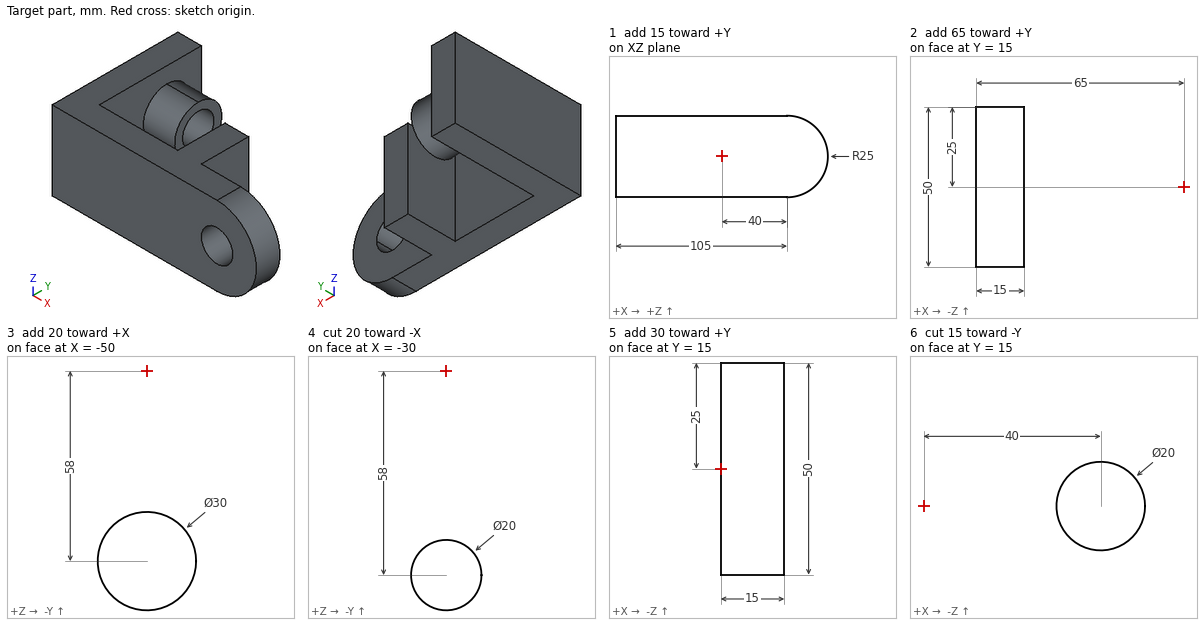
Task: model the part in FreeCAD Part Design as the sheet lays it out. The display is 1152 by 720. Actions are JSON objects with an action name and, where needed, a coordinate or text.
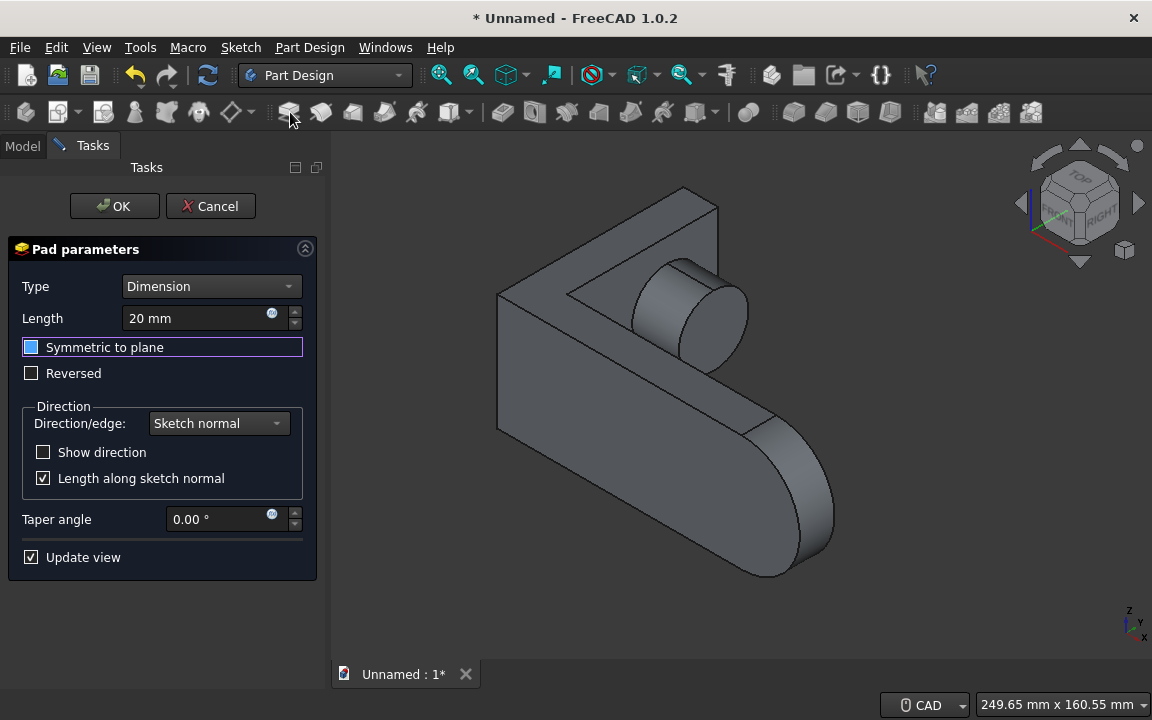
{"action": "left_click", "coordinate": [115, 206]}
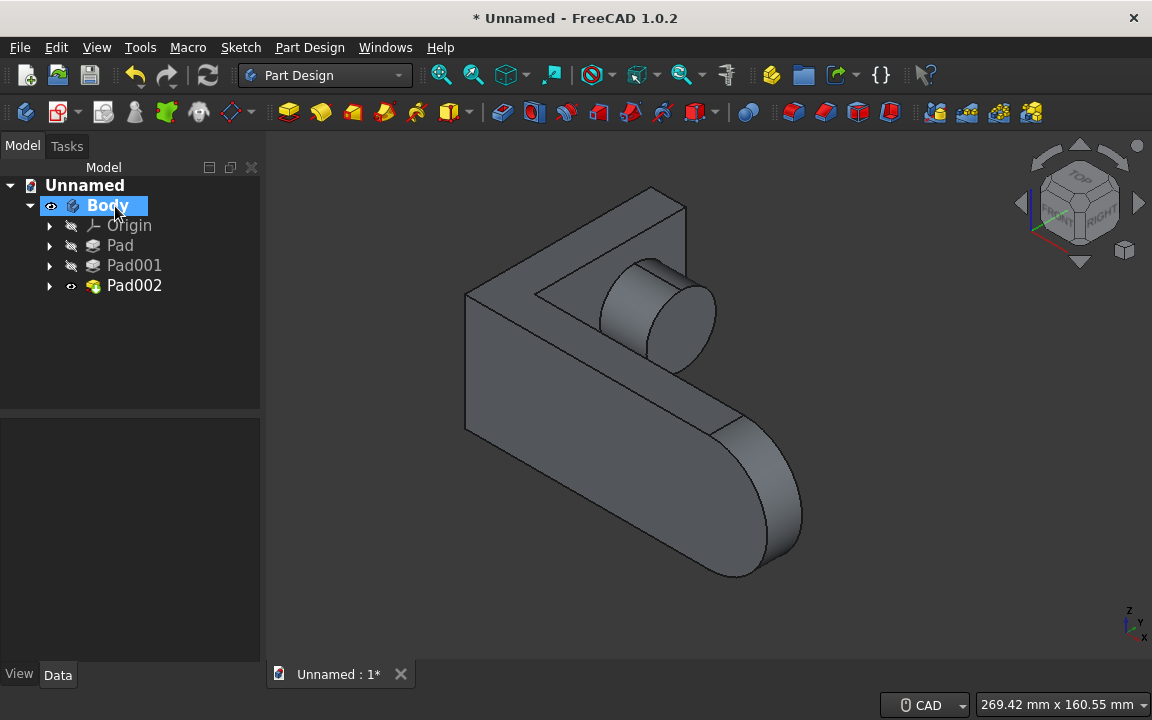
{"action": "left_click", "coordinate": [681, 330]}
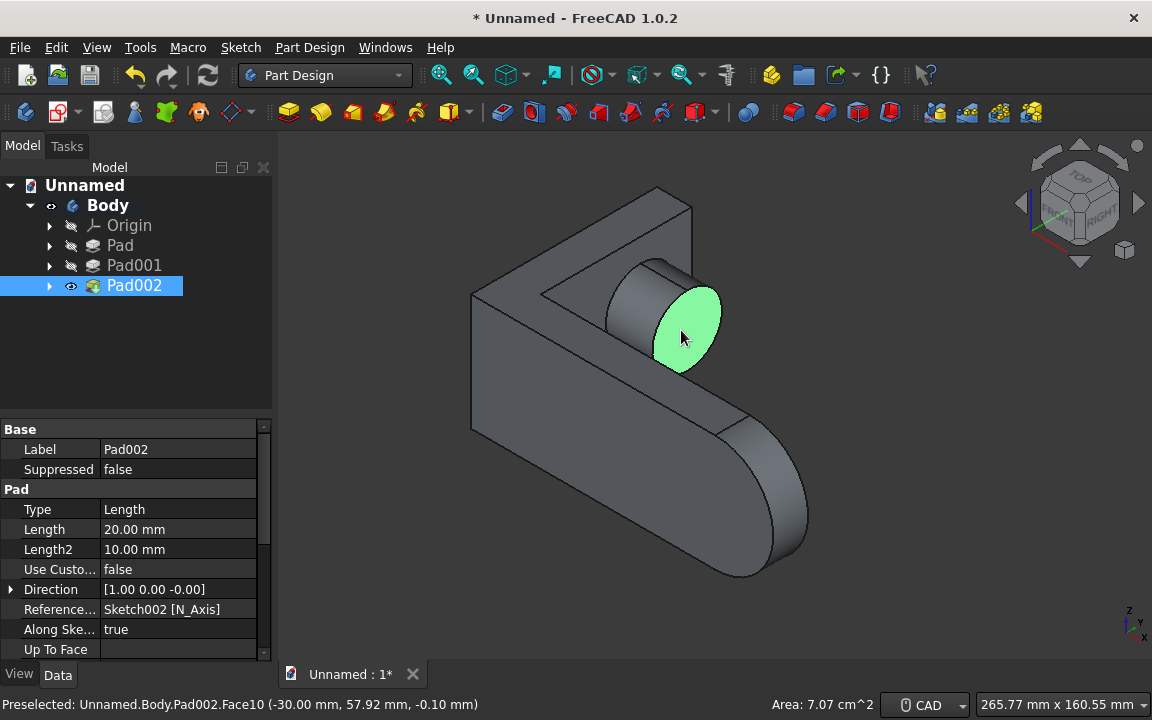
{"action": "left_click", "coordinate": [58, 112]}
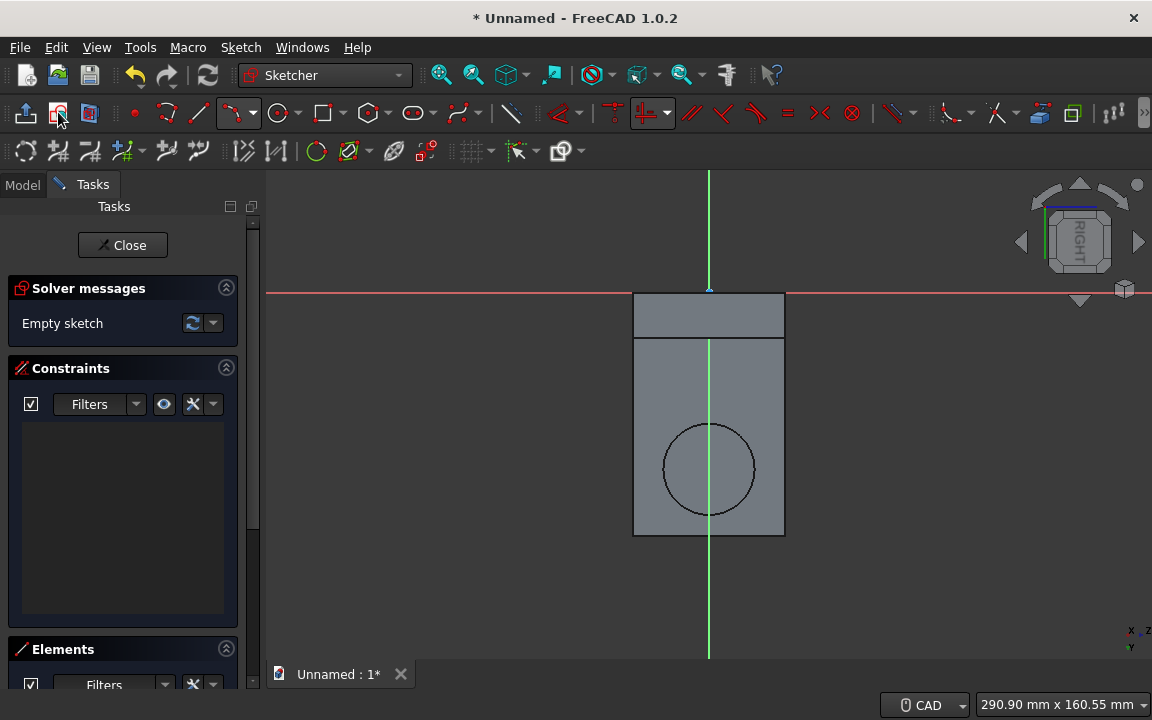
{"action": "left_click", "coordinate": [90, 114]}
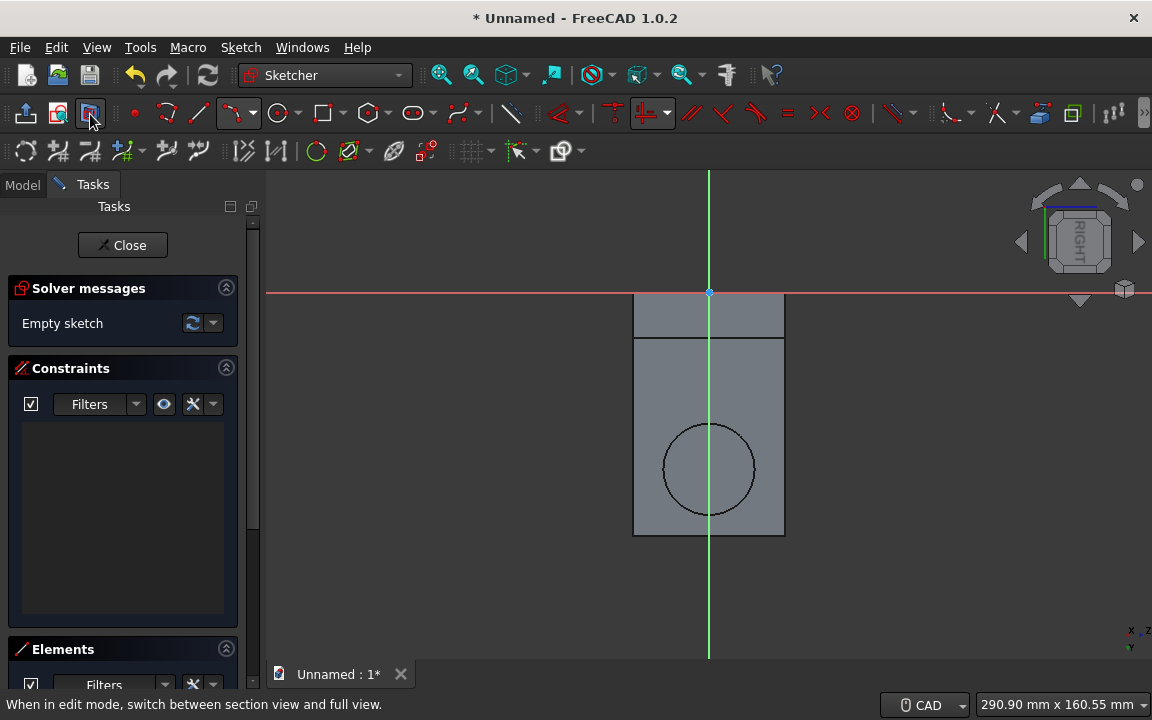
{"action": "scroll", "coordinate": [726, 483], "scroll_direction": "up", "scroll_amount": 8}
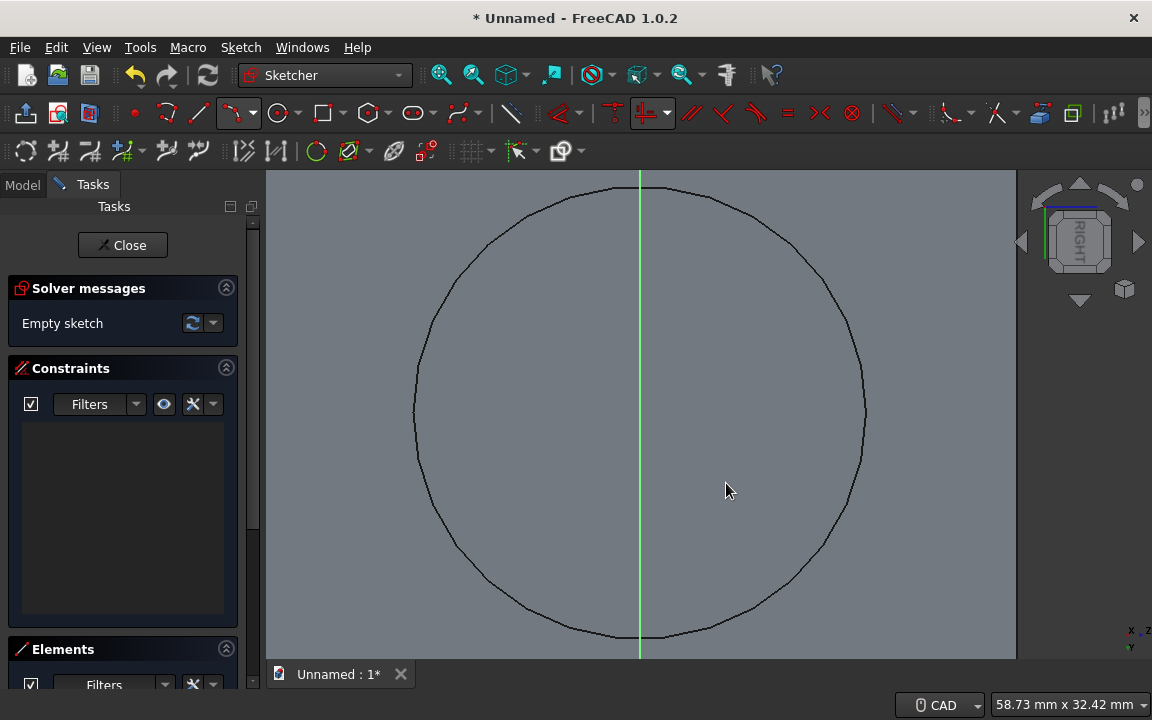
{"action": "left_click", "coordinate": [278, 114]}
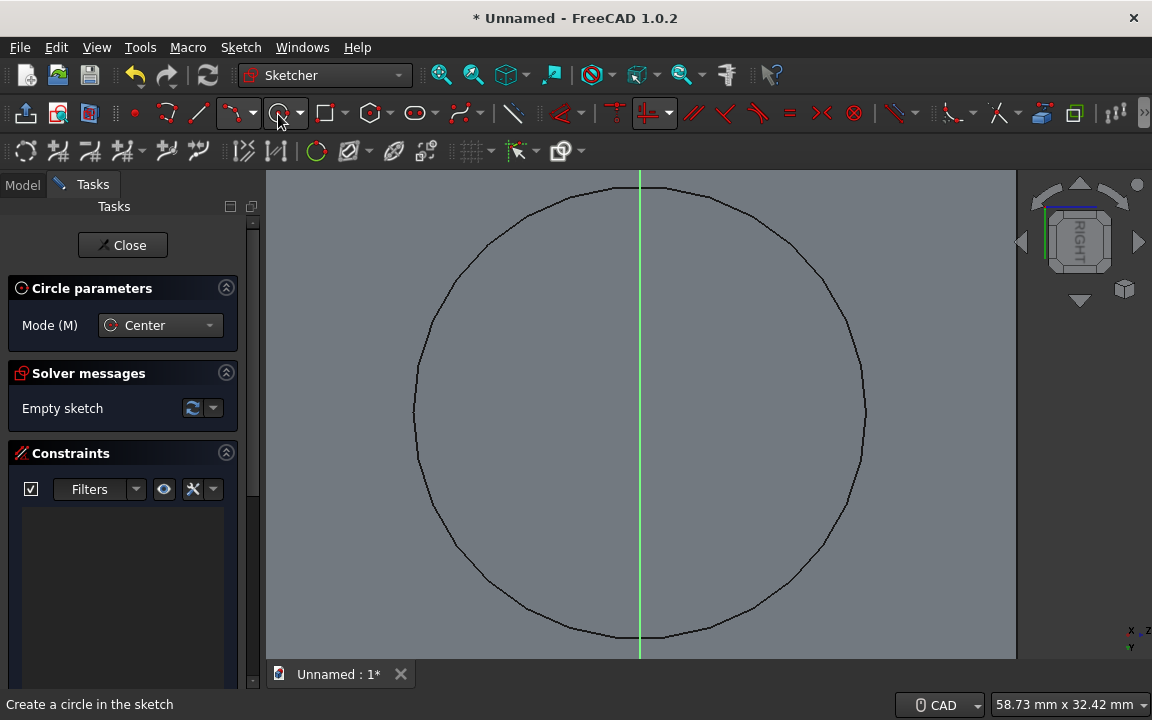
{"action": "left_click", "coordinate": [640, 413]}
{"action": "mouse_move", "coordinate": [746, 306]}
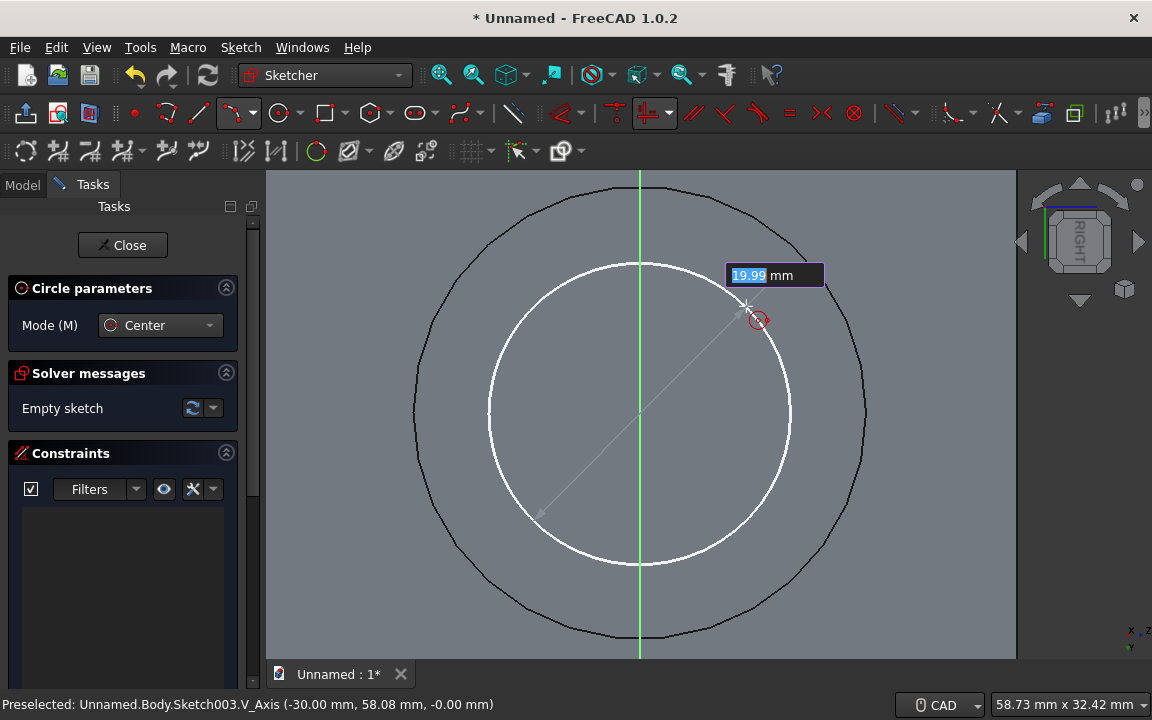
{"action": "type", "text": "20"}
{"action": "key", "text": "Return"}
{"action": "key", "text": "Escape"}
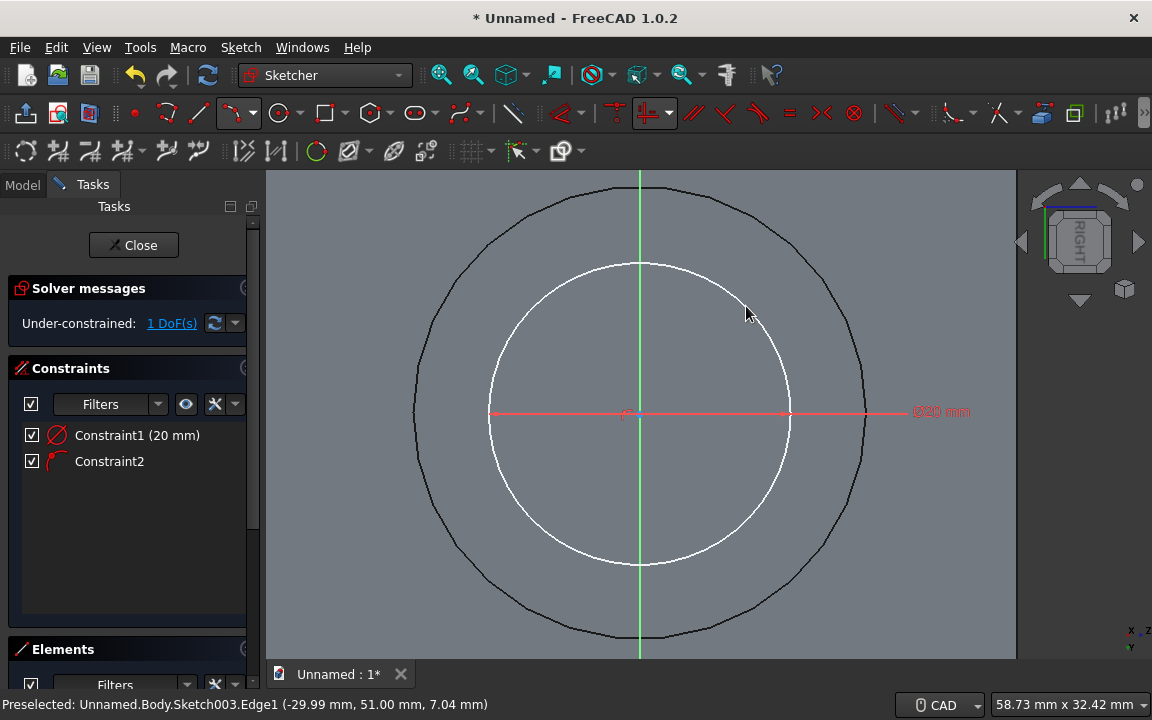
{"action": "left_click", "coordinate": [560, 114]}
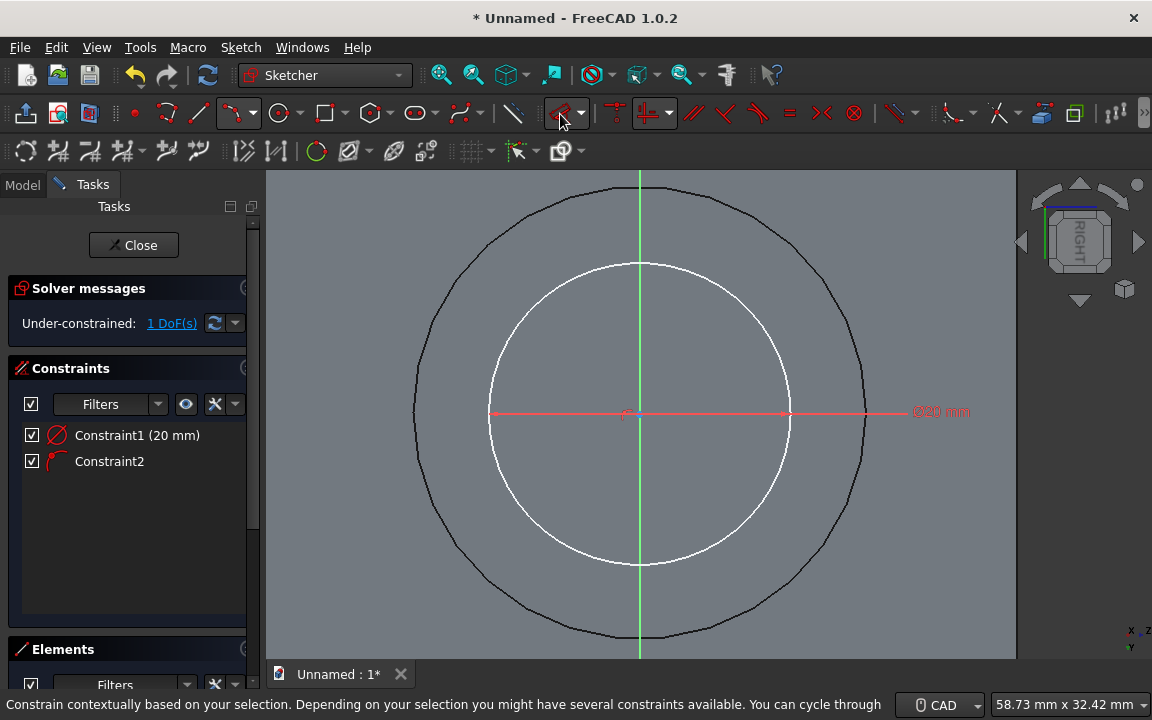
{"action": "left_click", "coordinate": [640, 414]}
{"action": "left_click", "coordinate": [674, 306]}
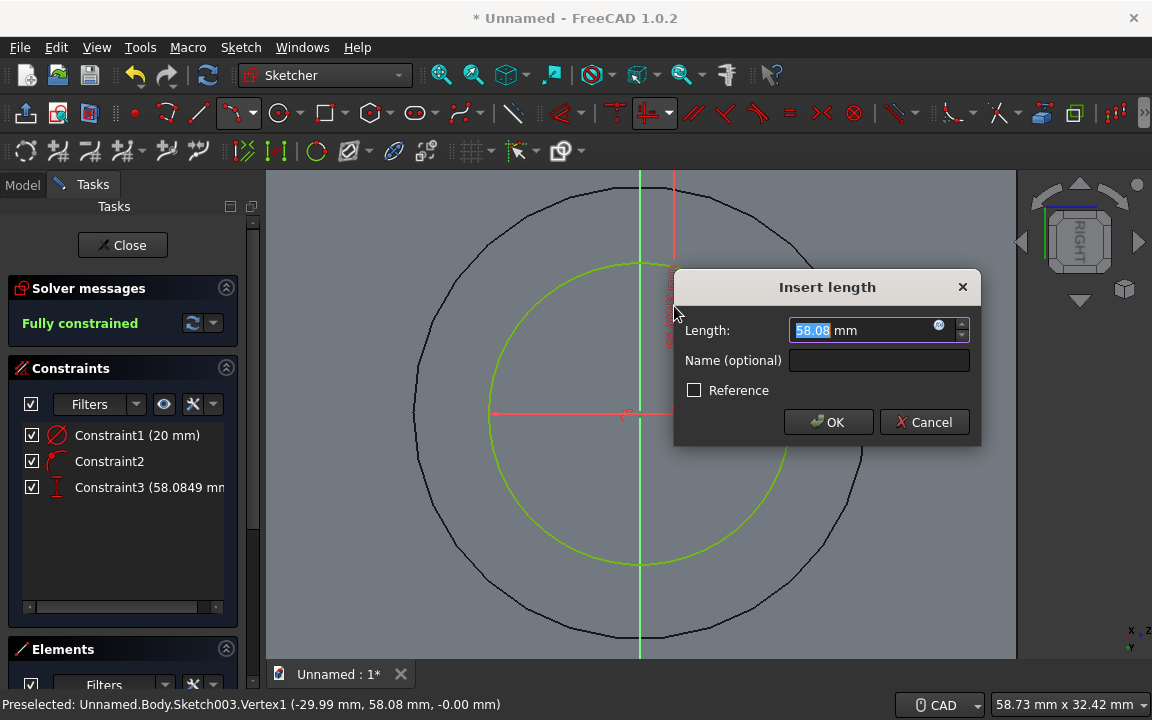
{"action": "type", "text": "58"}
{"action": "key", "text": "Return"}
{"action": "key", "text": "Escape"}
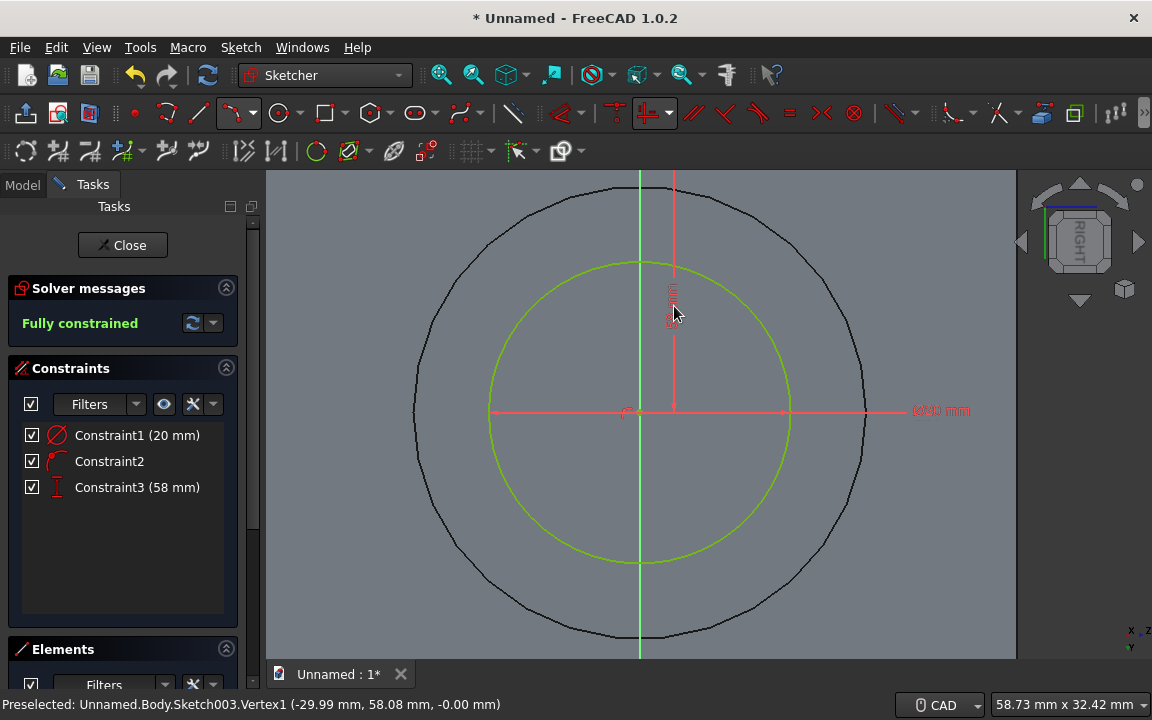
{"action": "left_click", "coordinate": [123, 245]}